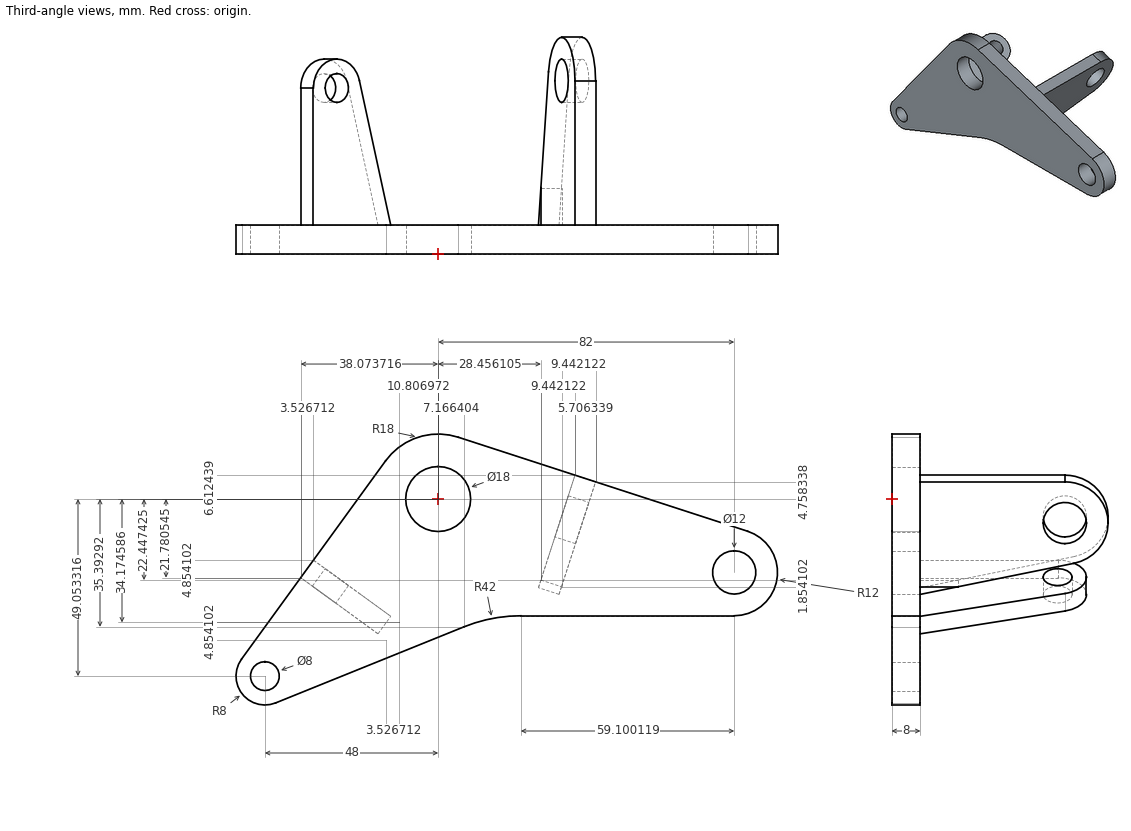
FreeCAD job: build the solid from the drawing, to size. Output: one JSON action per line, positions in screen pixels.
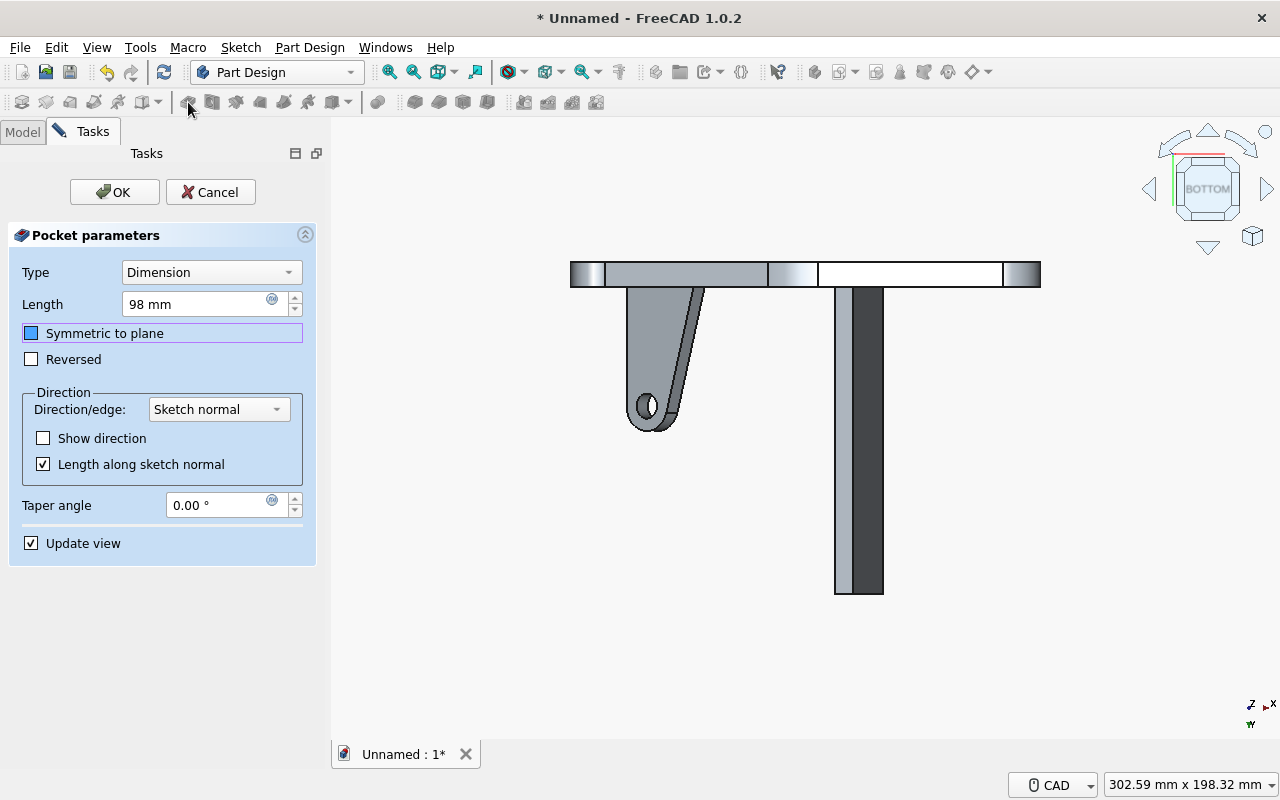
{"action": "left_click", "coordinate": [115, 192]}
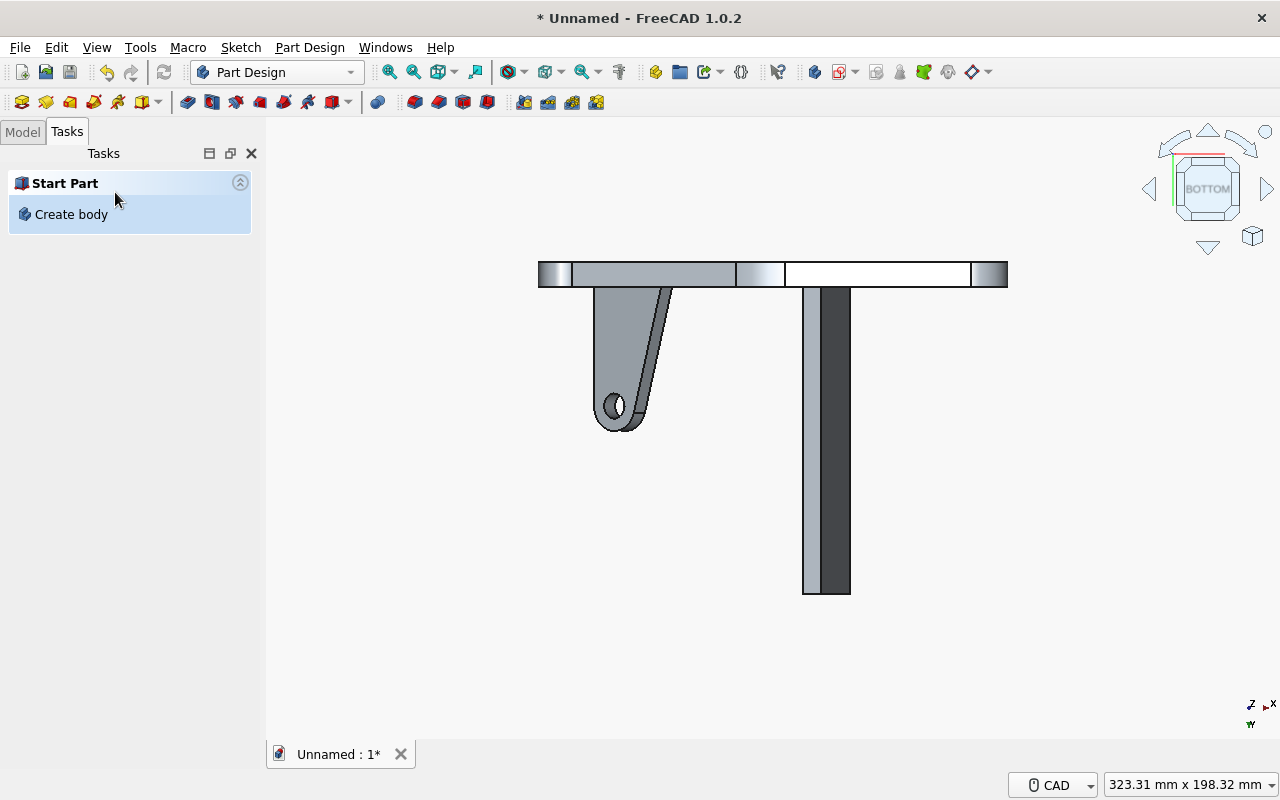
{"action": "left_click", "coordinate": [835, 352]}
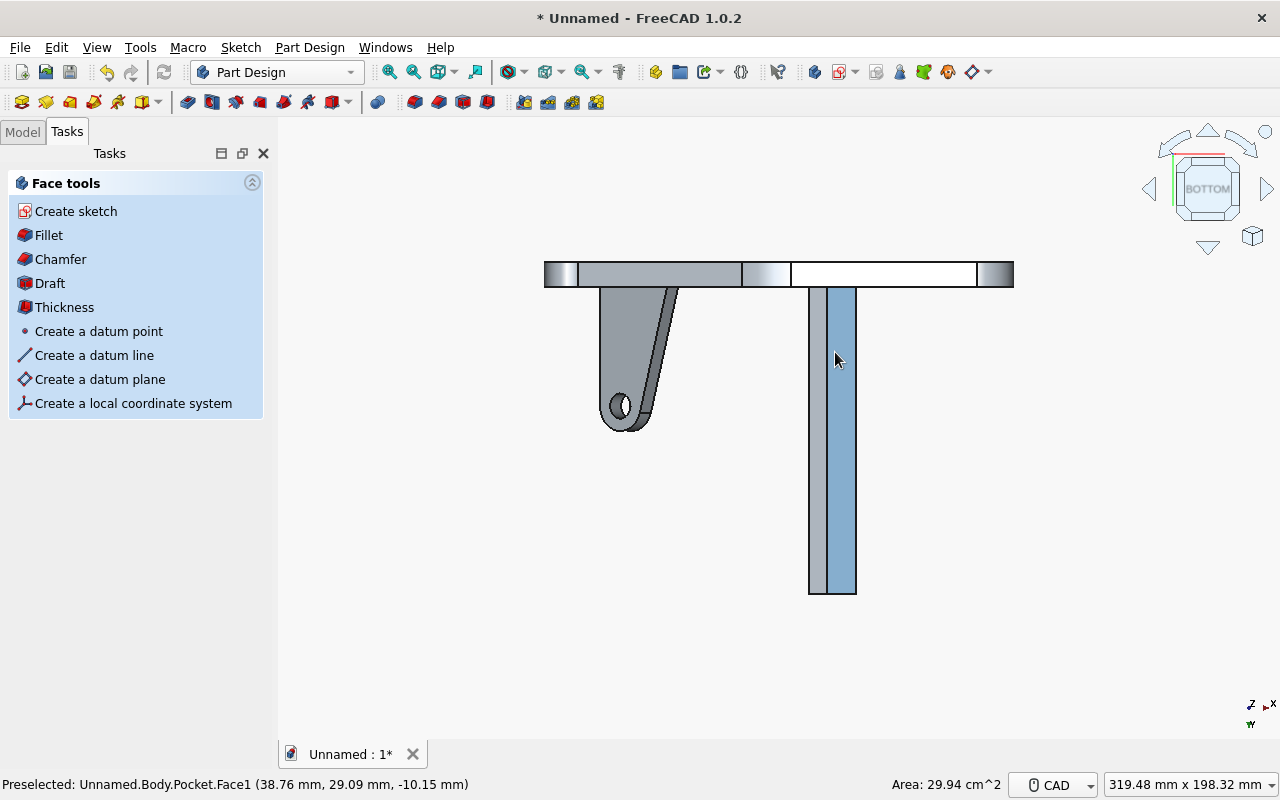
{"action": "left_click", "coordinate": [840, 72]}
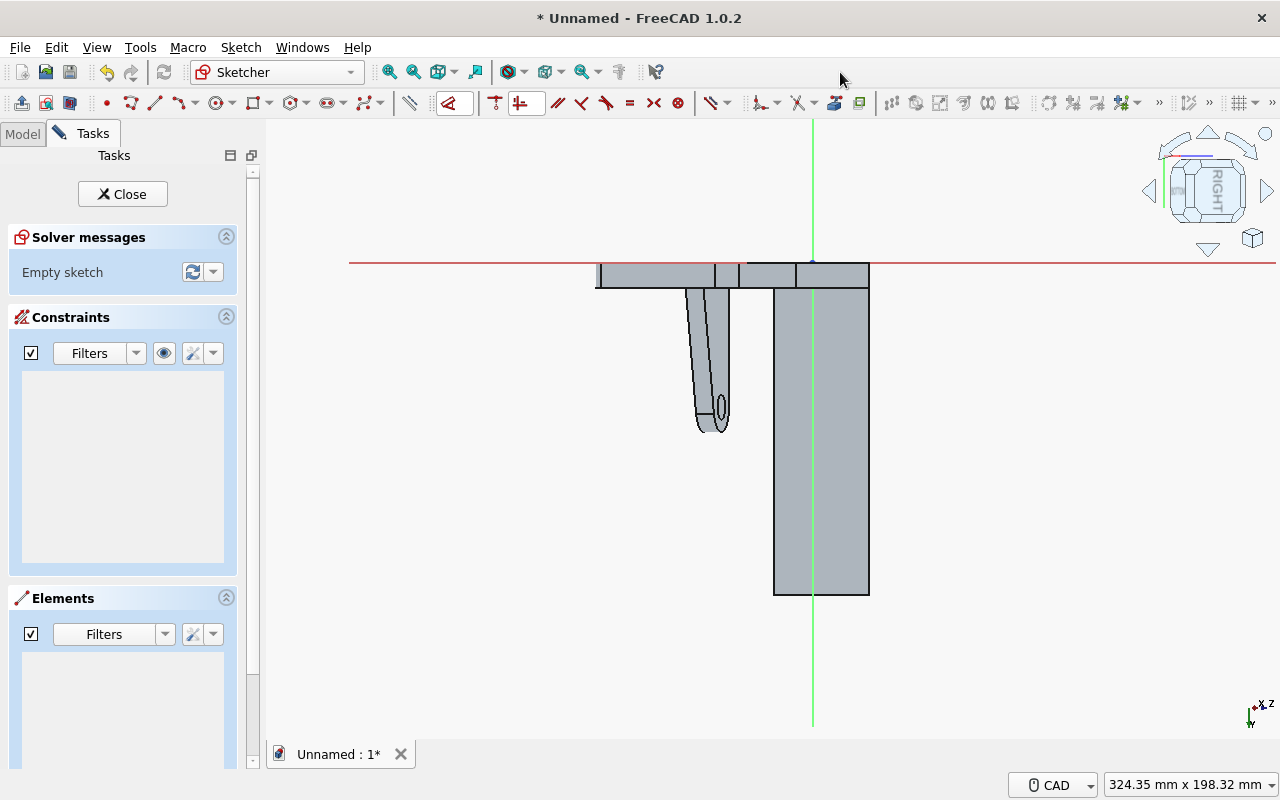
{"action": "left_click", "coordinate": [70, 104]}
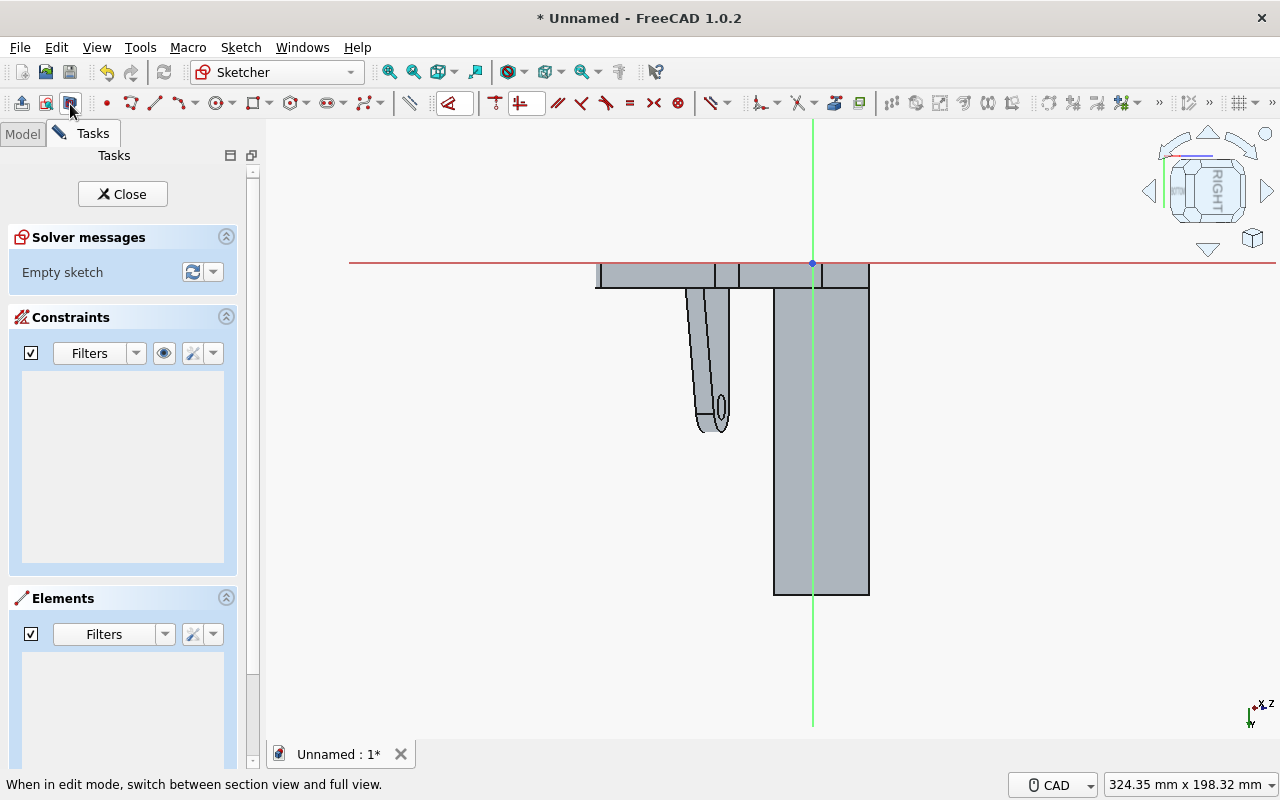
{"action": "scroll", "coordinate": [910, 298], "scroll_direction": "up", "scroll_amount": 4}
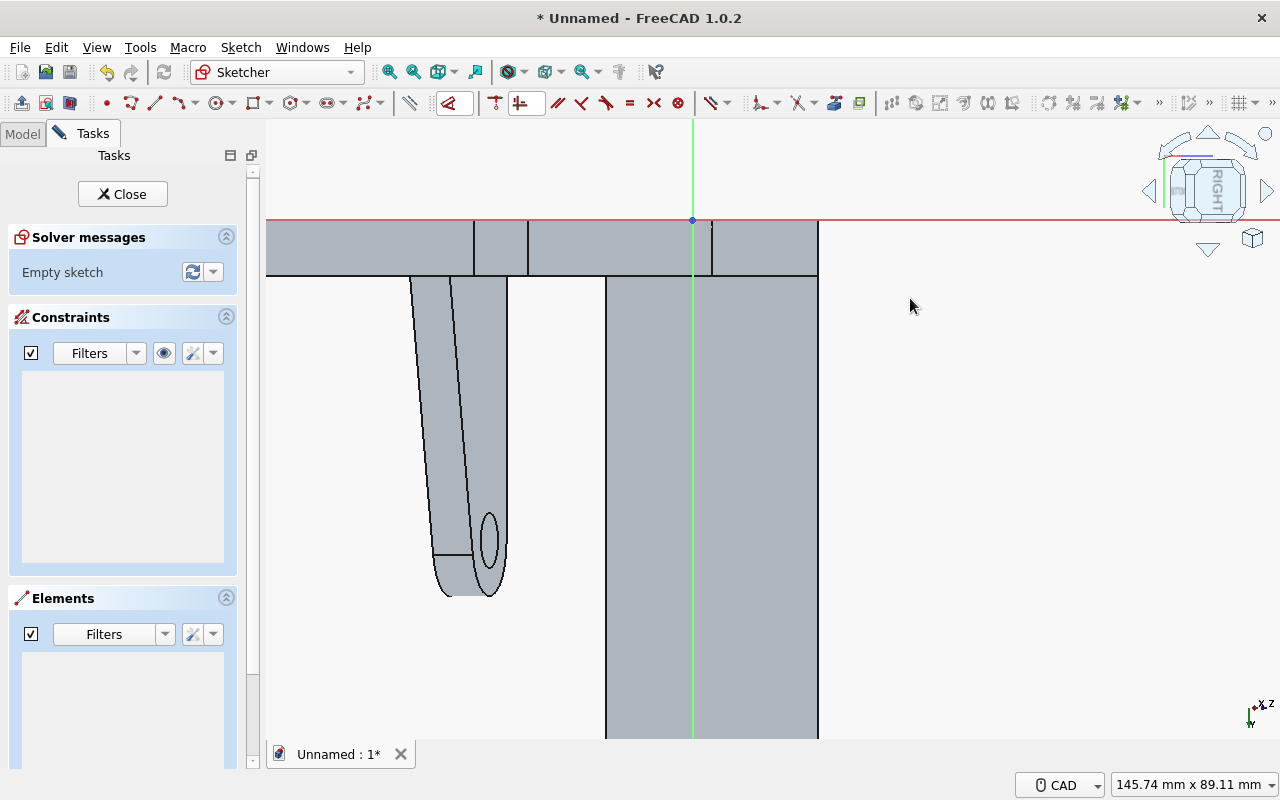
{"action": "left_click", "coordinate": [132, 104]}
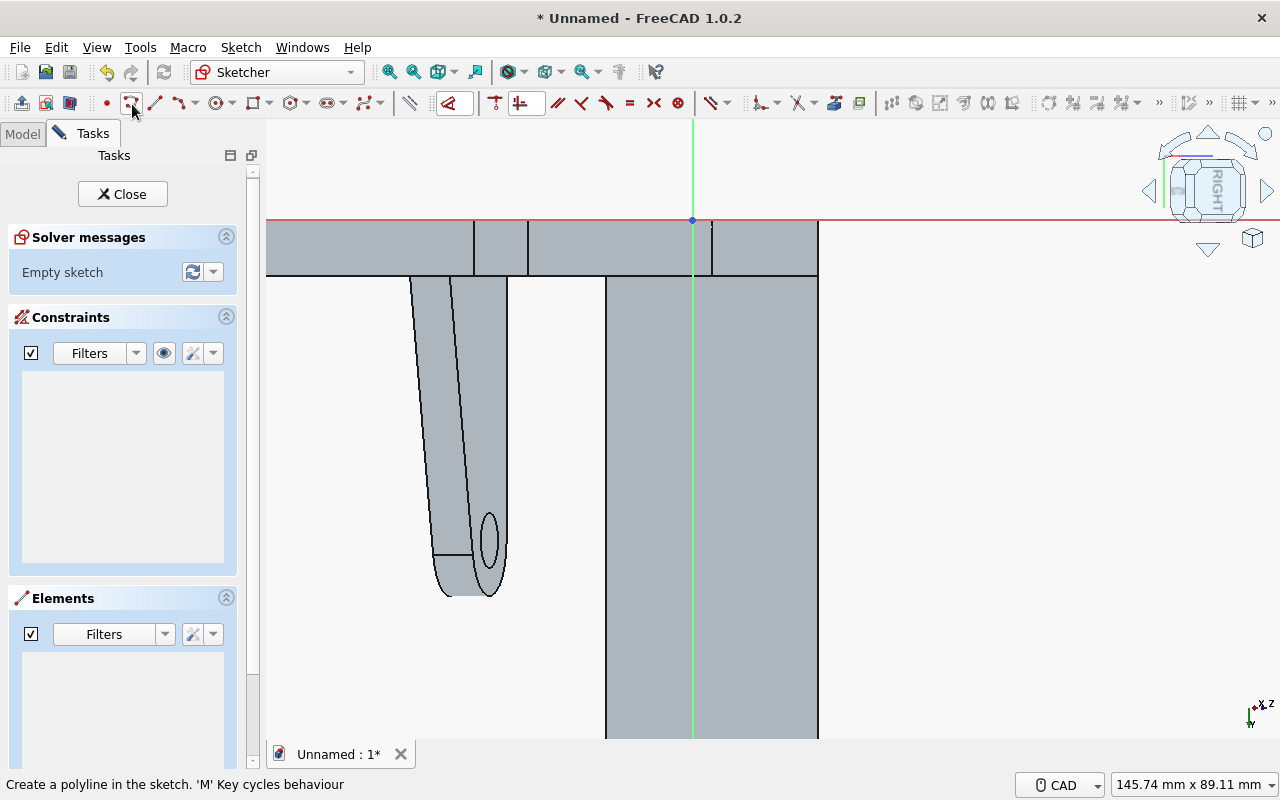
{"action": "left_click", "coordinate": [818, 554]}
{"action": "left_click", "coordinate": [818, 276]}
{"action": "left_click", "coordinate": [590, 276]}
{"action": "left_click", "coordinate": [653, 572]}
{"action": "right_click", "coordinate": [653, 572]}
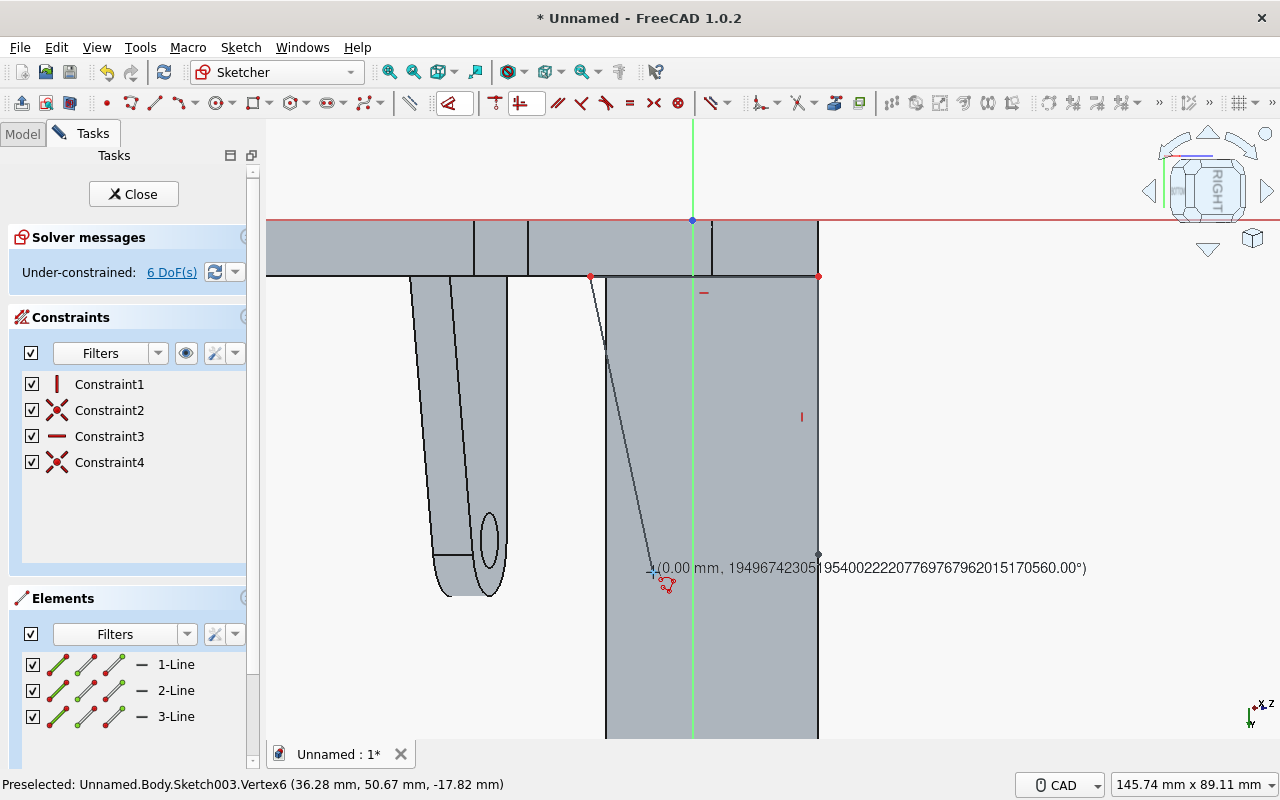
{"action": "key", "text": "g 3 a"}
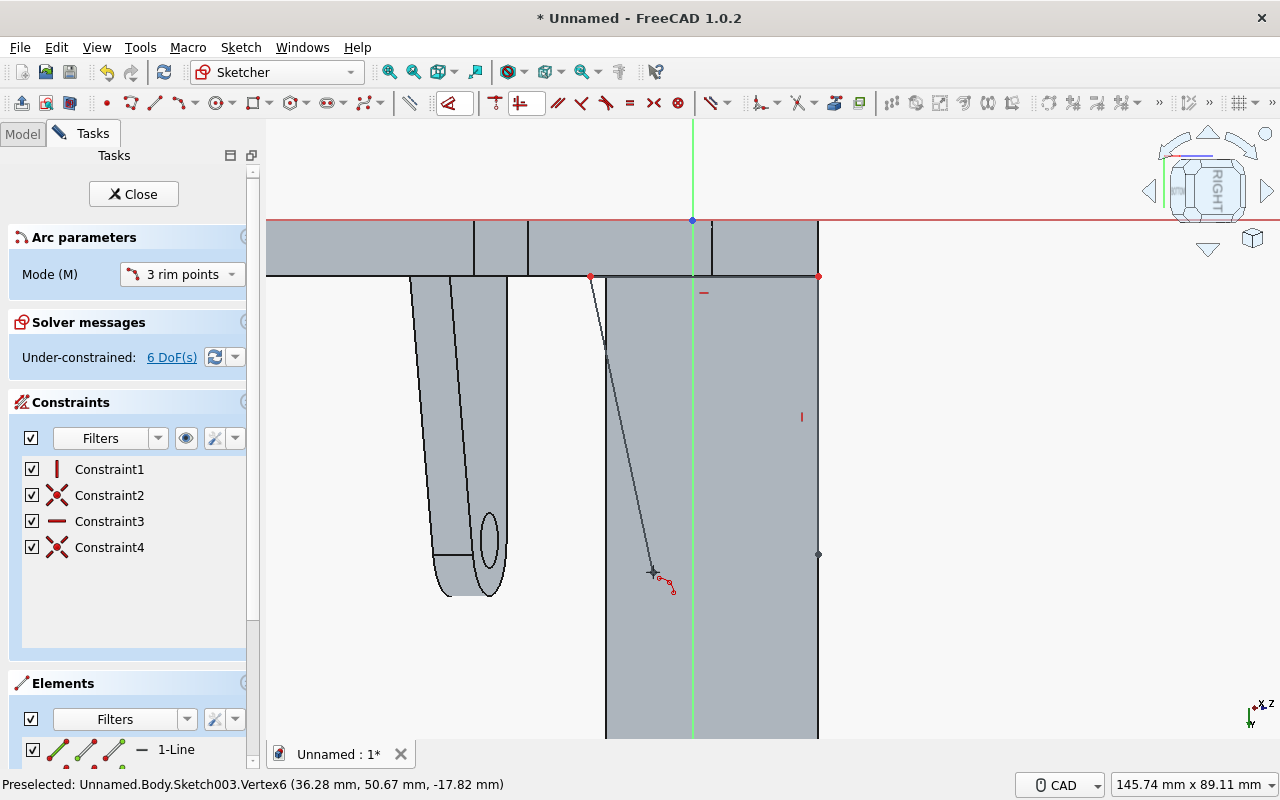
{"action": "left_click", "coordinate": [653, 573]}
{"action": "left_click", "coordinate": [818, 555]}
{"action": "left_click", "coordinate": [743, 637]}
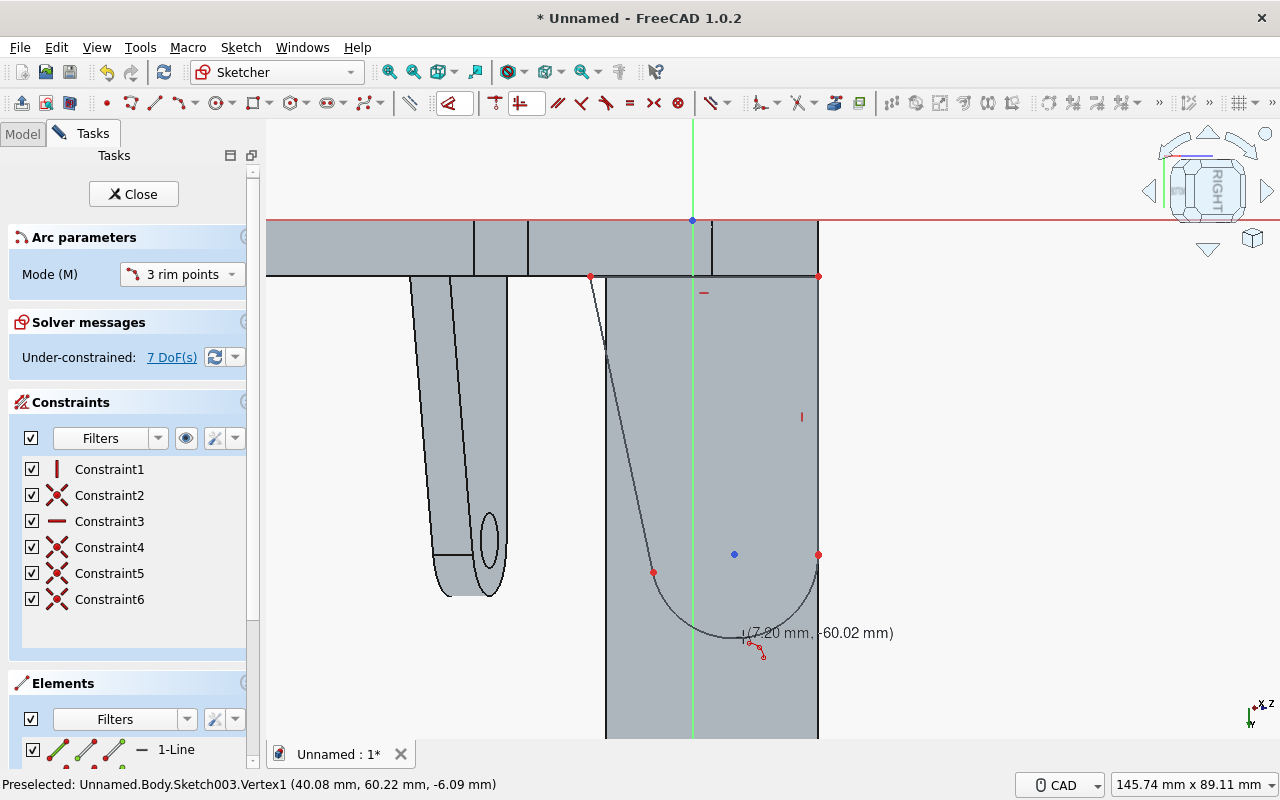
{"action": "left_click", "coordinate": [216, 104]}